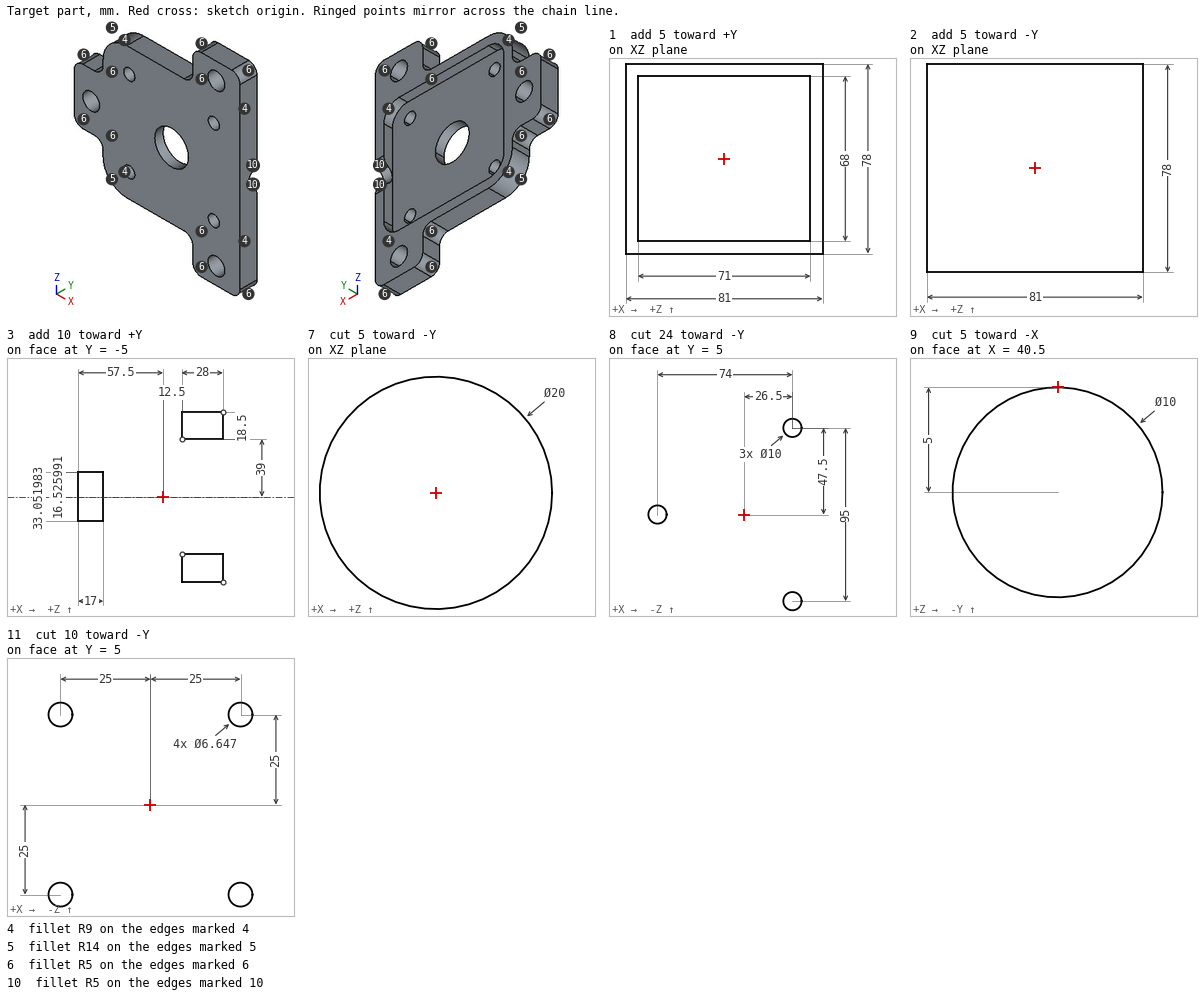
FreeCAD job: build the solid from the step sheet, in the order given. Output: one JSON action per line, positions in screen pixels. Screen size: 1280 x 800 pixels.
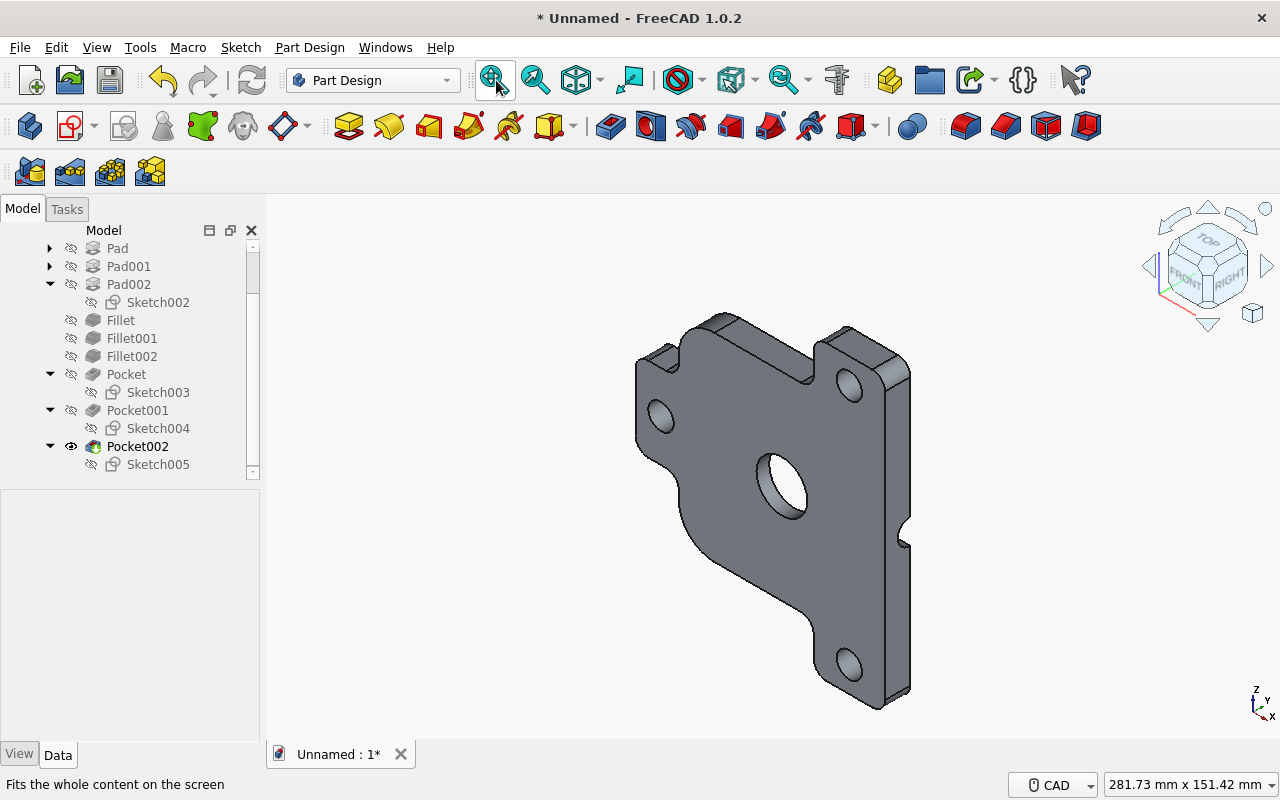
{"action": "key", "text": "1"}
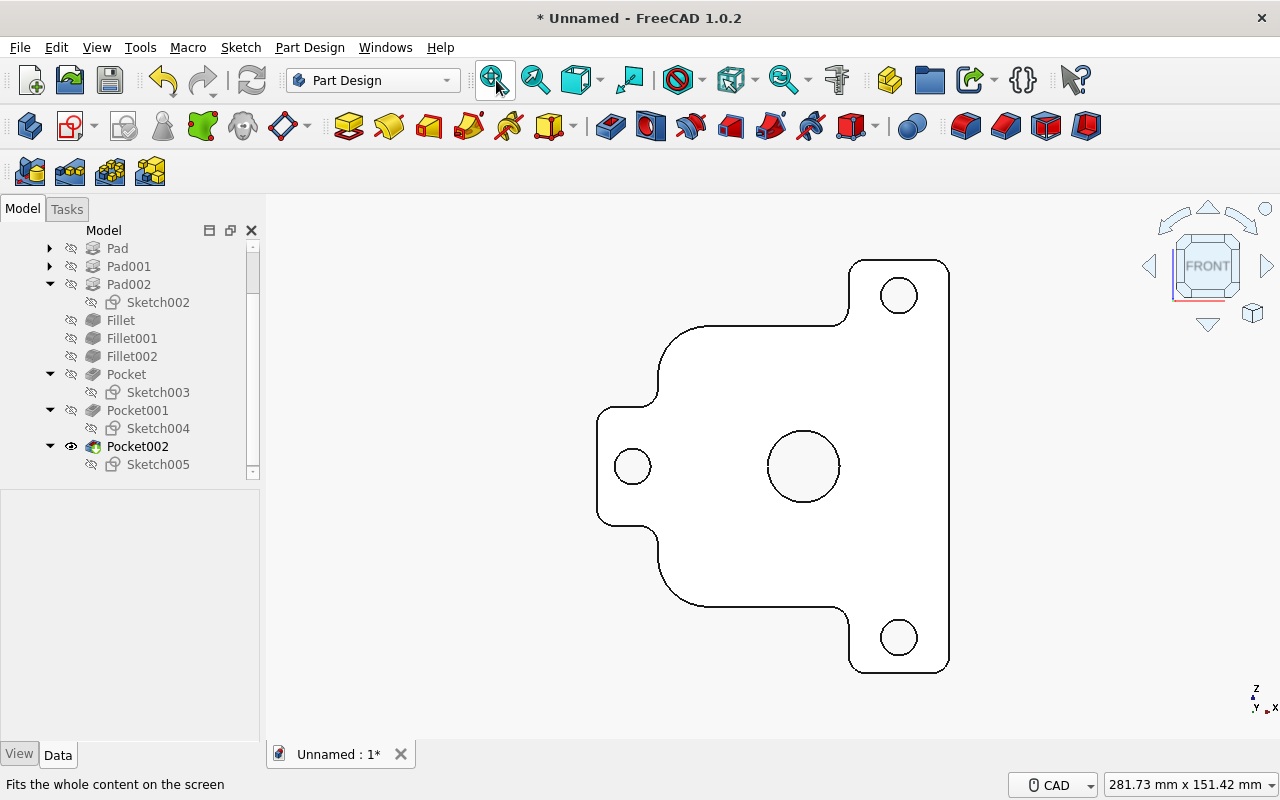
{"action": "scroll", "coordinate": [940, 448], "scroll_direction": "up", "scroll_amount": 4}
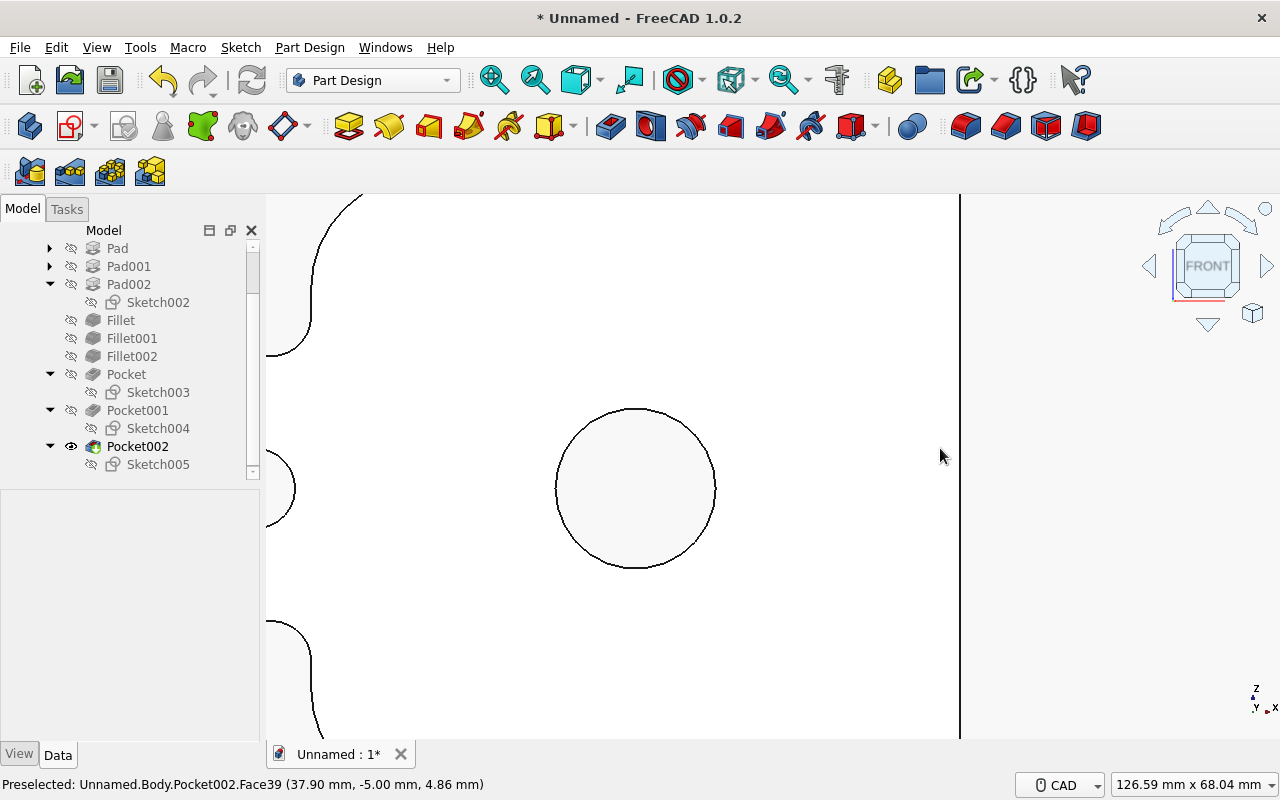
{"action": "key", "text": "v f"}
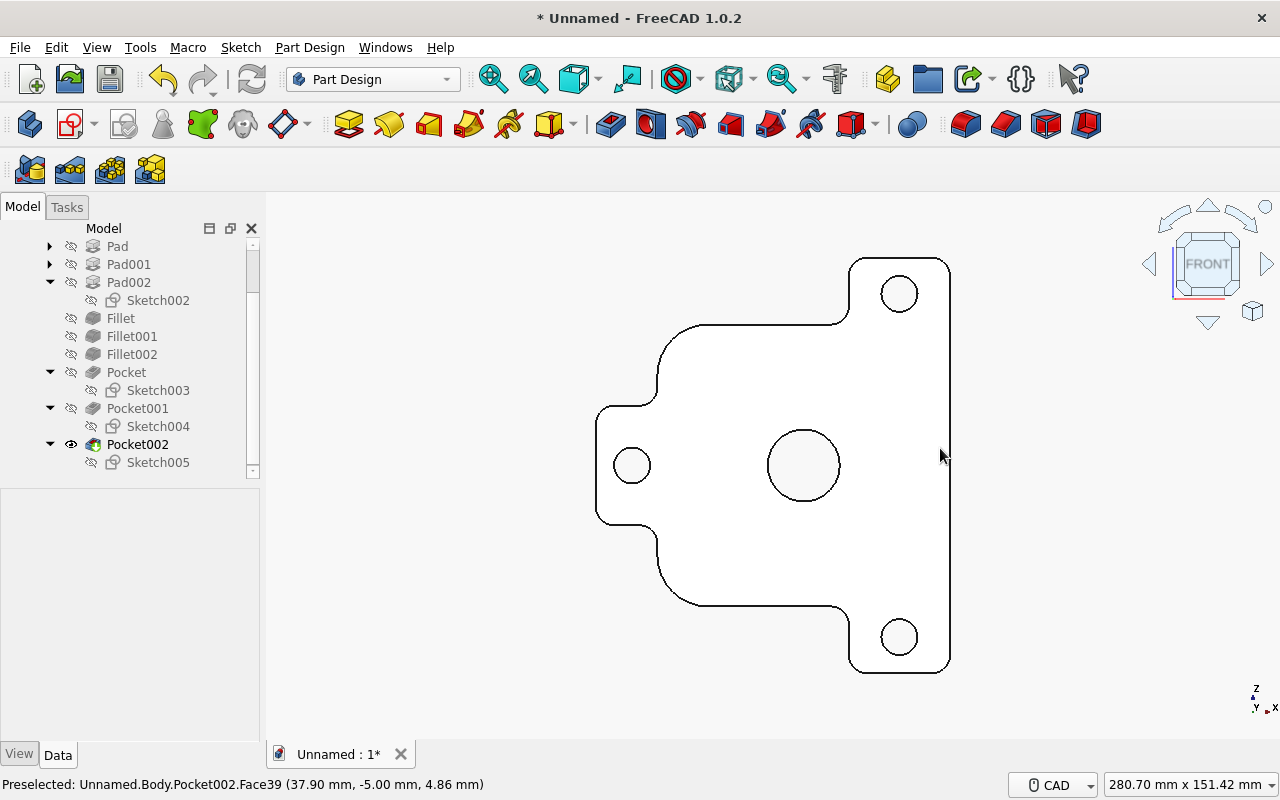
{"action": "key", "text": "3"}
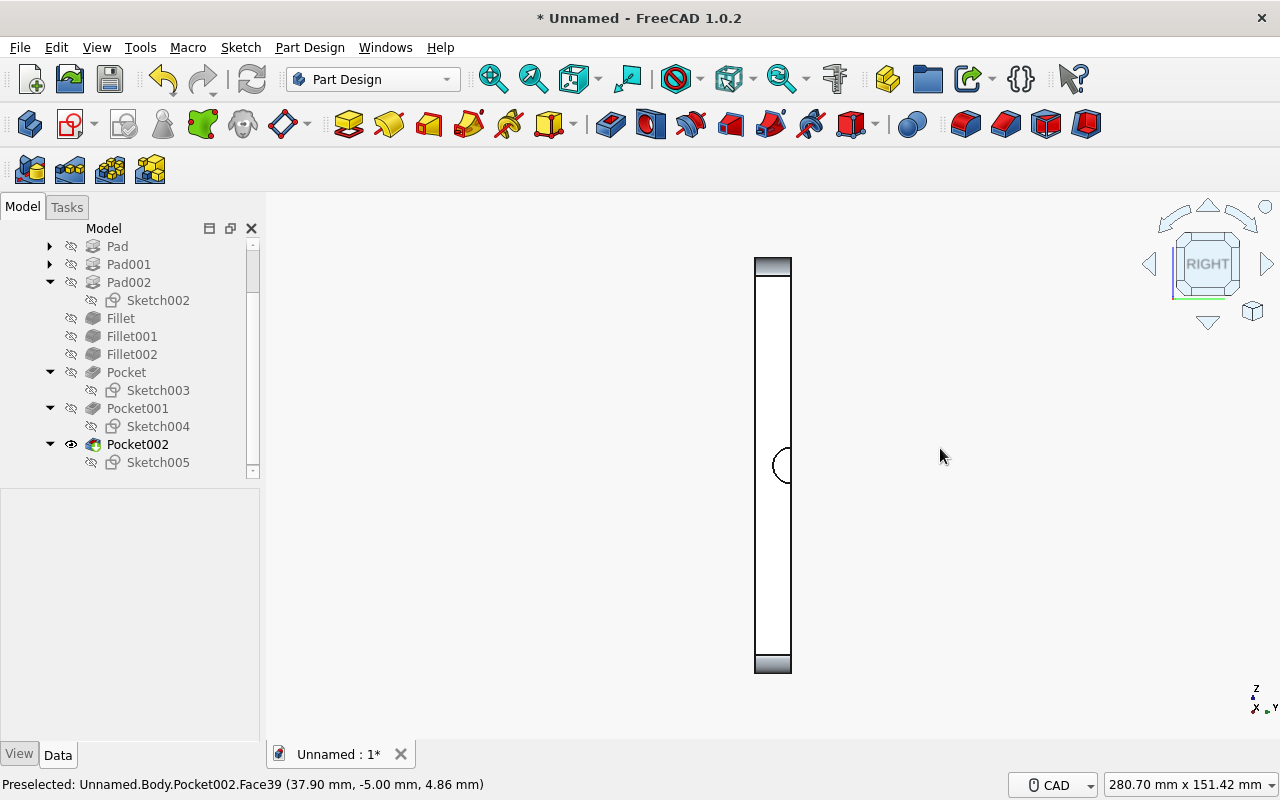
{"action": "scroll", "coordinate": [791, 446], "scroll_direction": "up", "scroll_amount": 4}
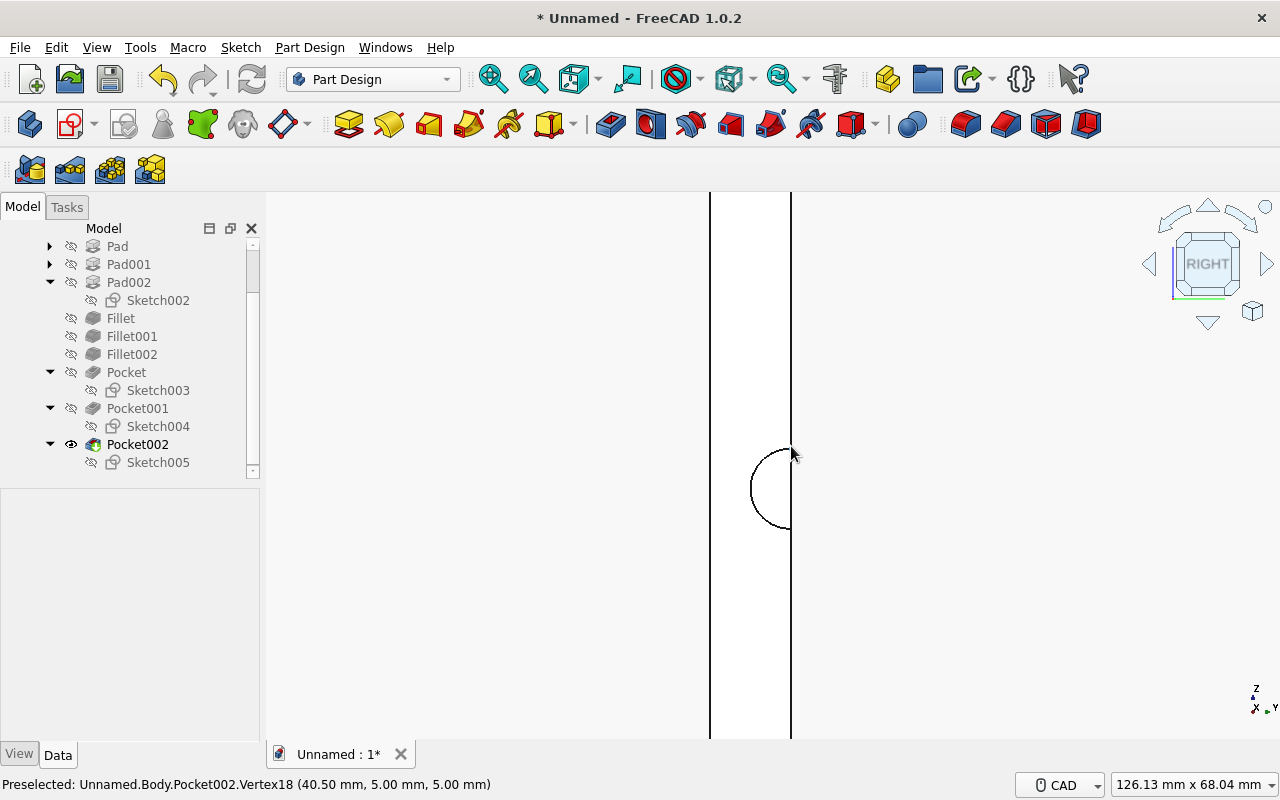
{"action": "left_click", "coordinate": [494, 80]}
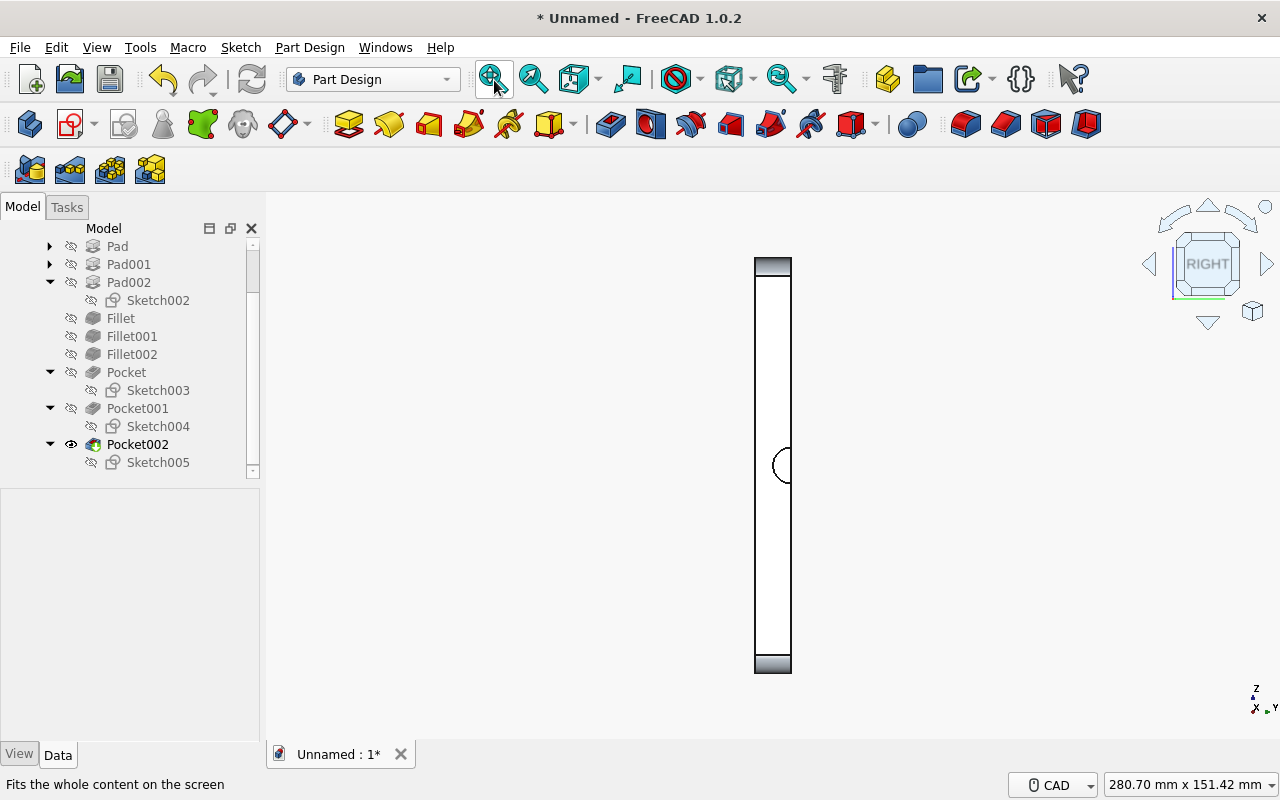
{"action": "key", "text": "5"}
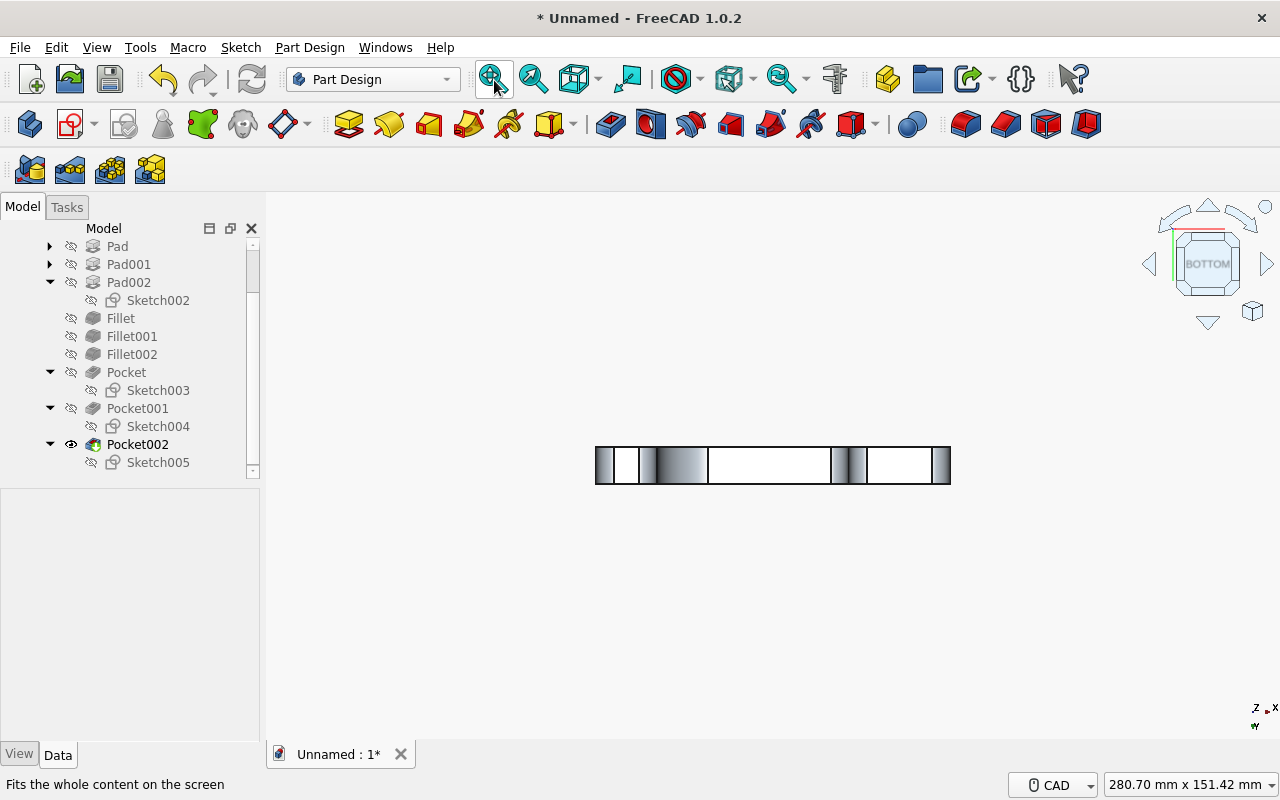
{"action": "key", "text": "v f"}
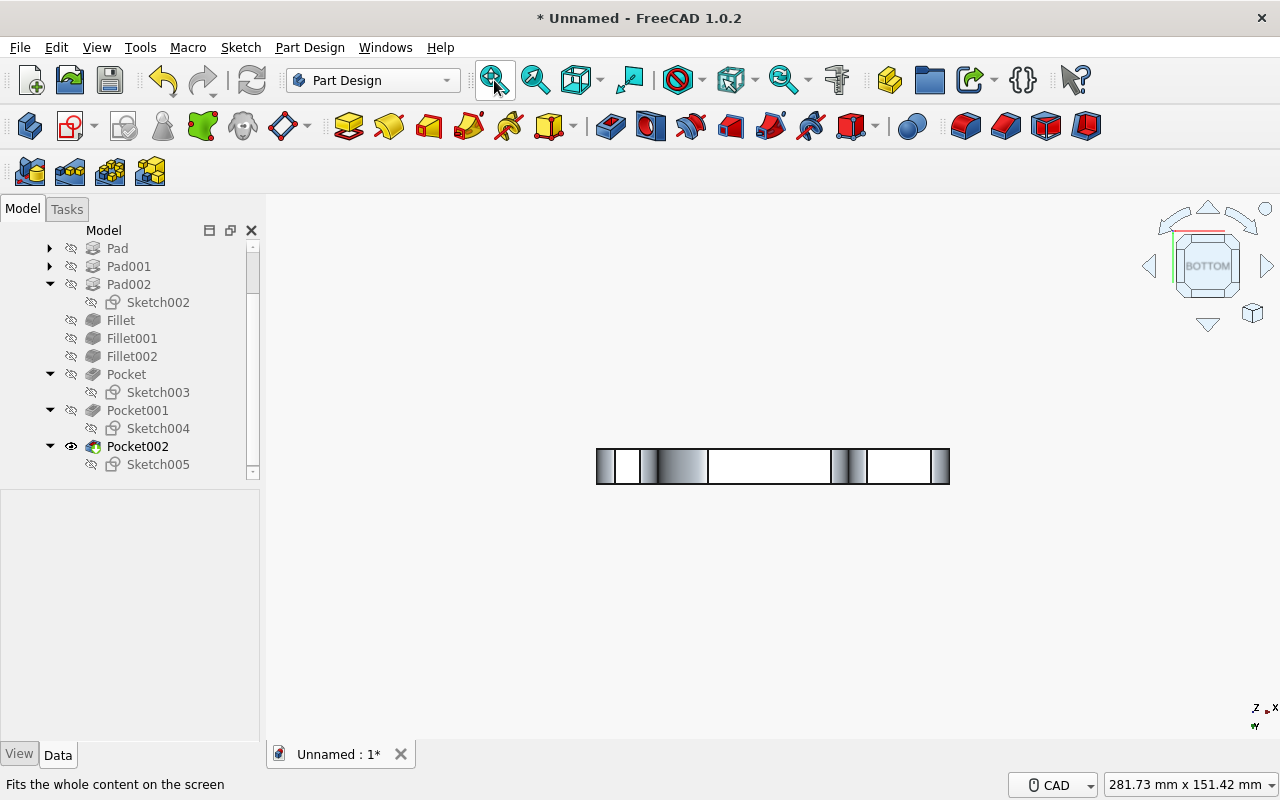
{"action": "scroll", "coordinate": [940, 483], "scroll_direction": "up", "scroll_amount": 4}